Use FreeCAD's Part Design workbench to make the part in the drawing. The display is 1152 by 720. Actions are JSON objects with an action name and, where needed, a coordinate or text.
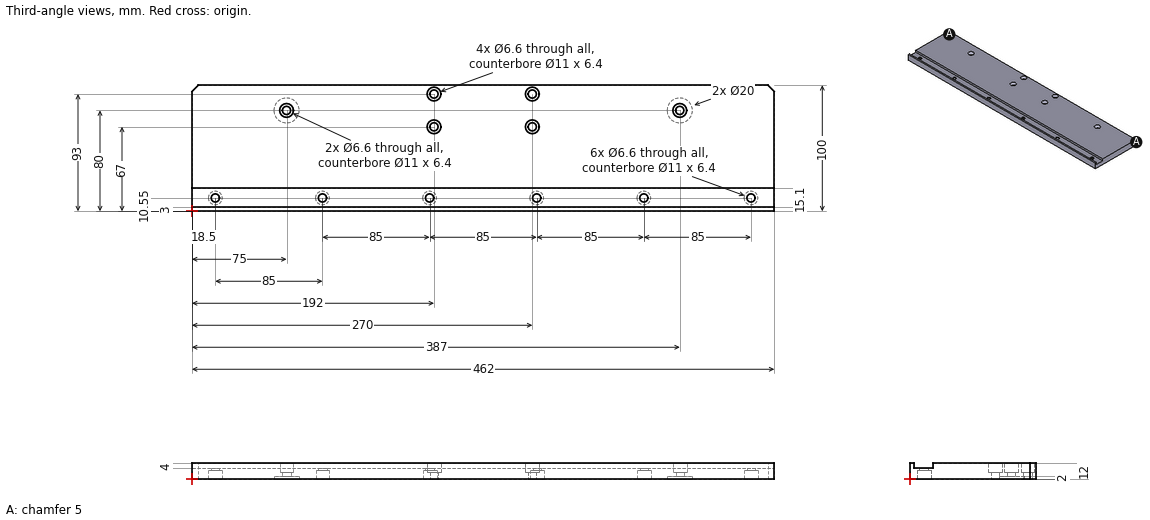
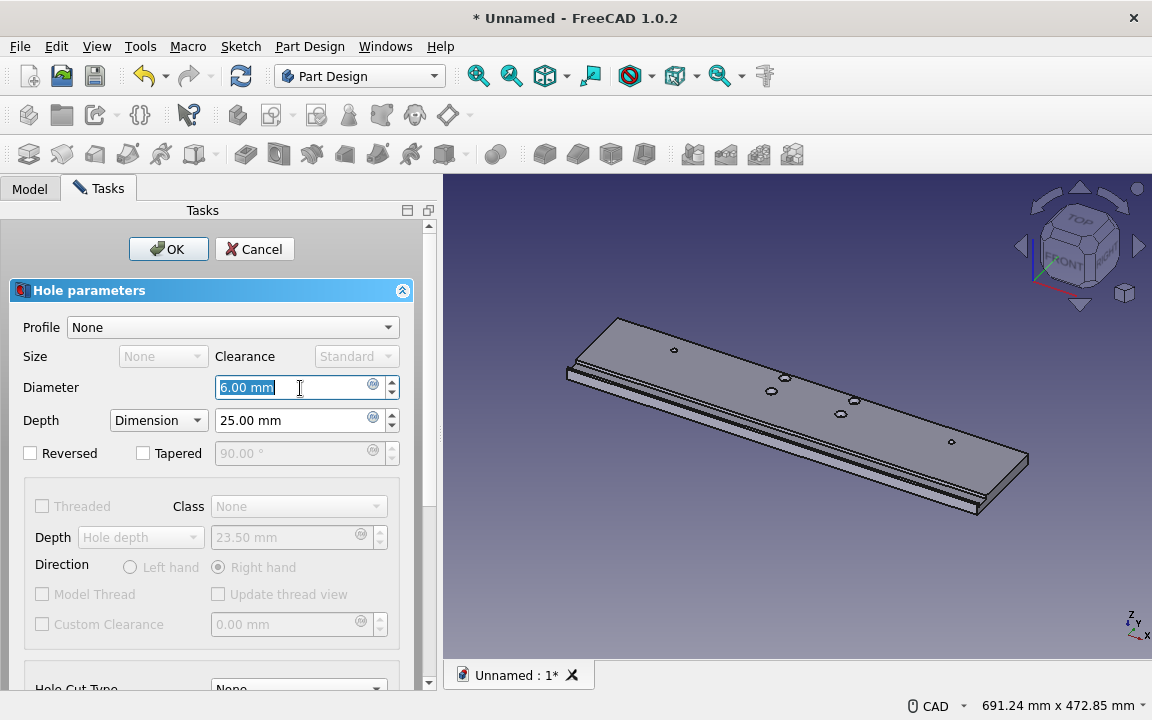
{"action": "type", "text": "6.6"}
{"action": "key", "text": "Tab"}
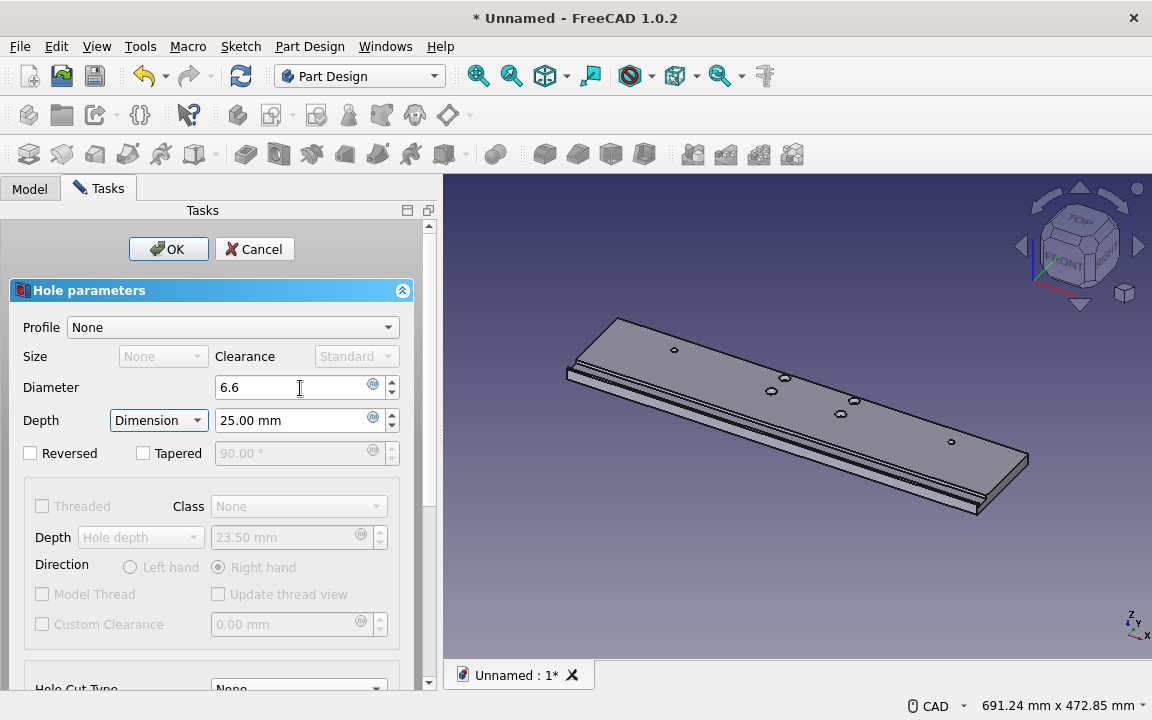
{"action": "left_click", "coordinate": [160, 420]}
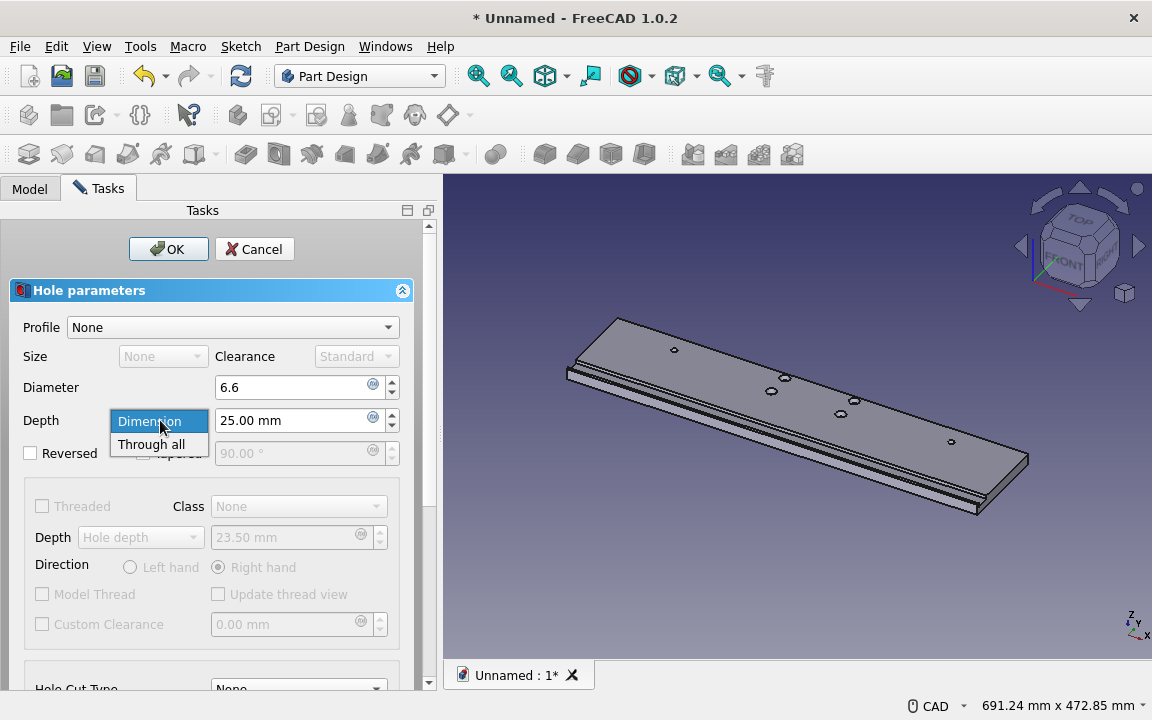
{"action": "left_click", "coordinate": [158, 444]}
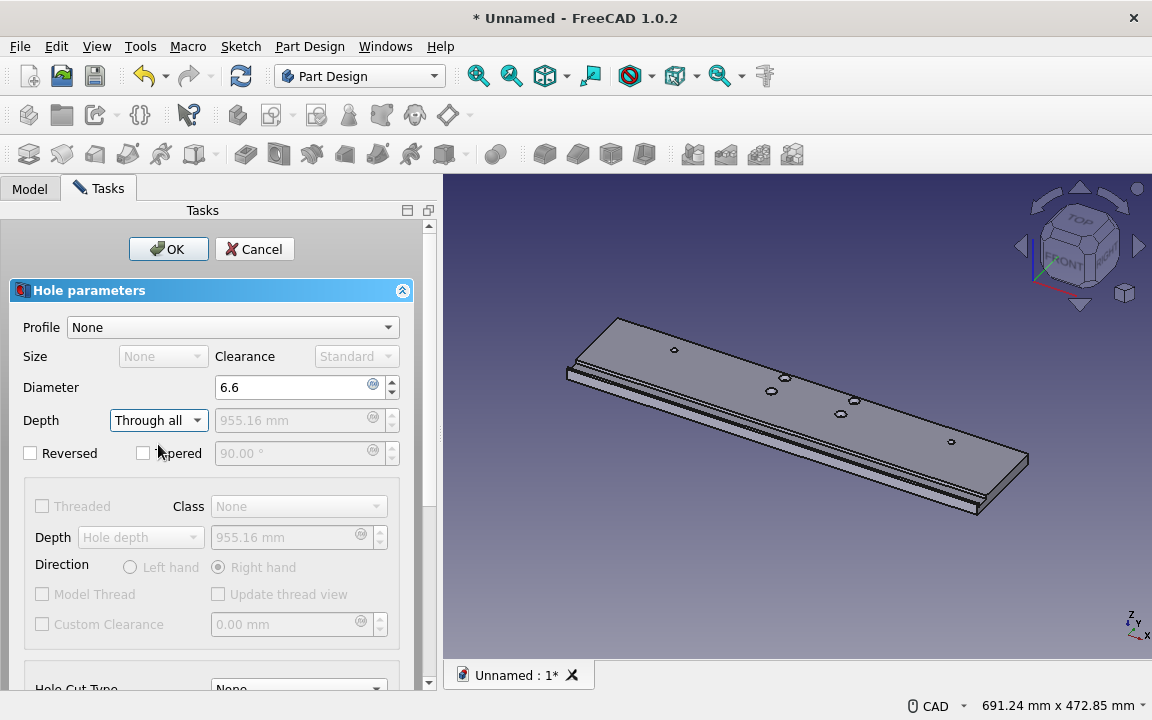
{"action": "scroll", "coordinate": [429, 455], "scroll_direction": "down", "scroll_amount": 2}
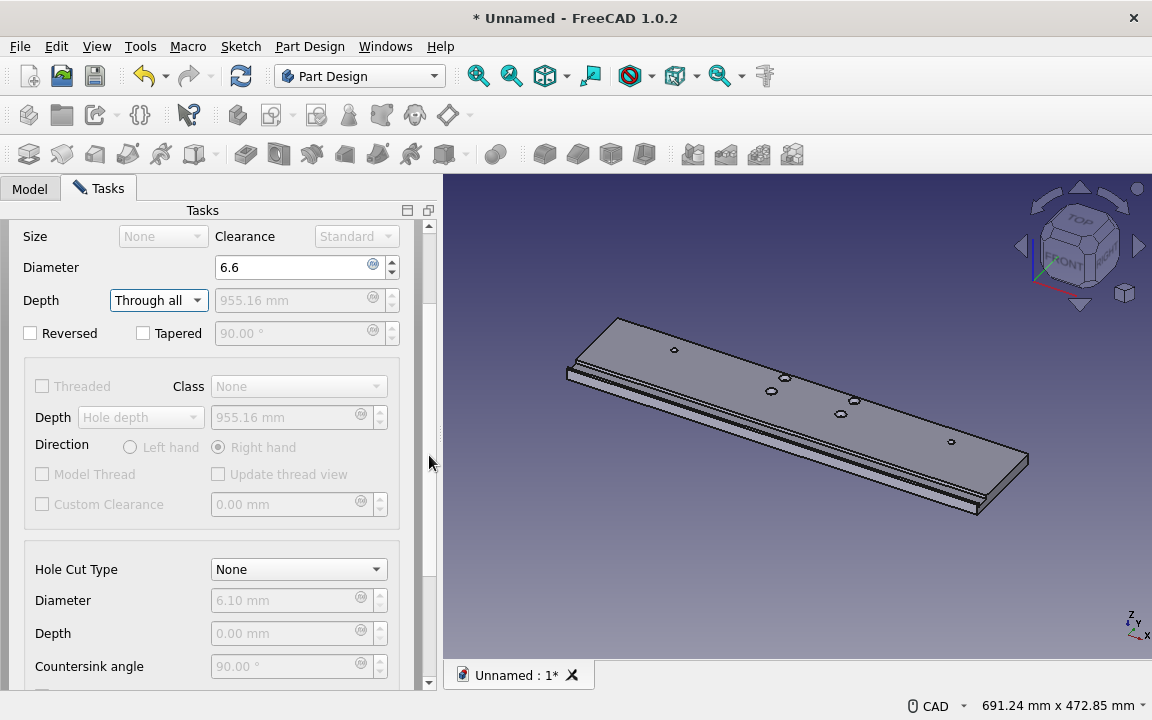
{"action": "left_click", "coordinate": [300, 570]}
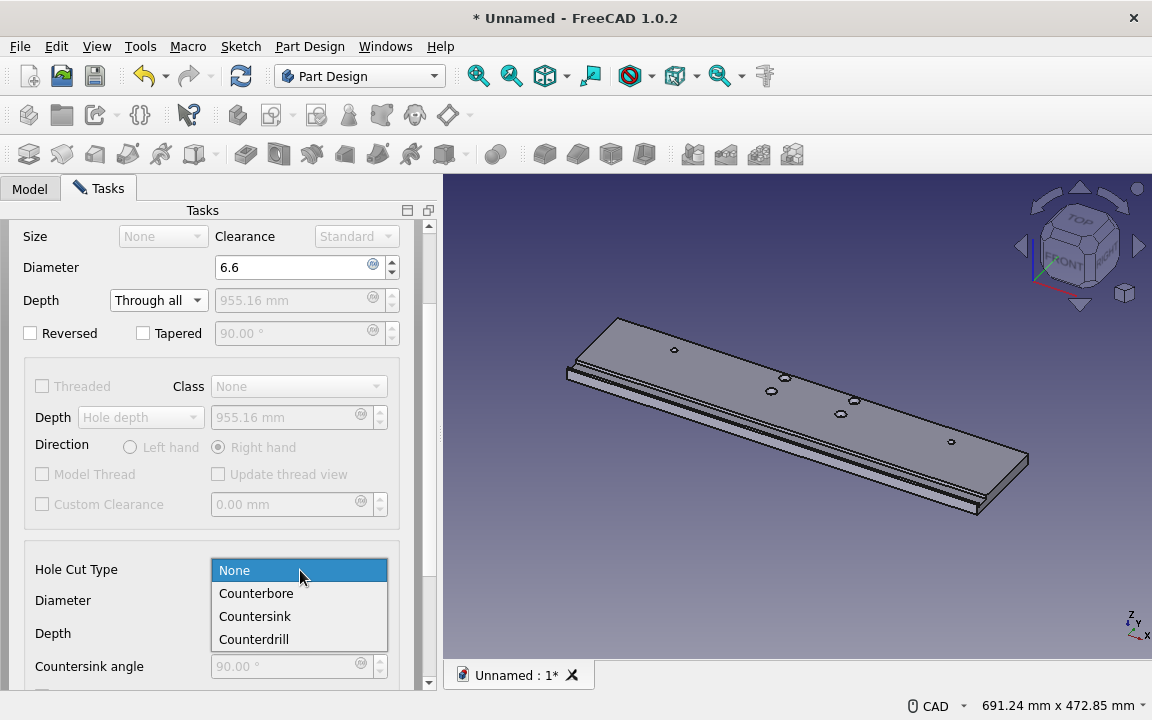
{"action": "left_click", "coordinate": [298, 594]}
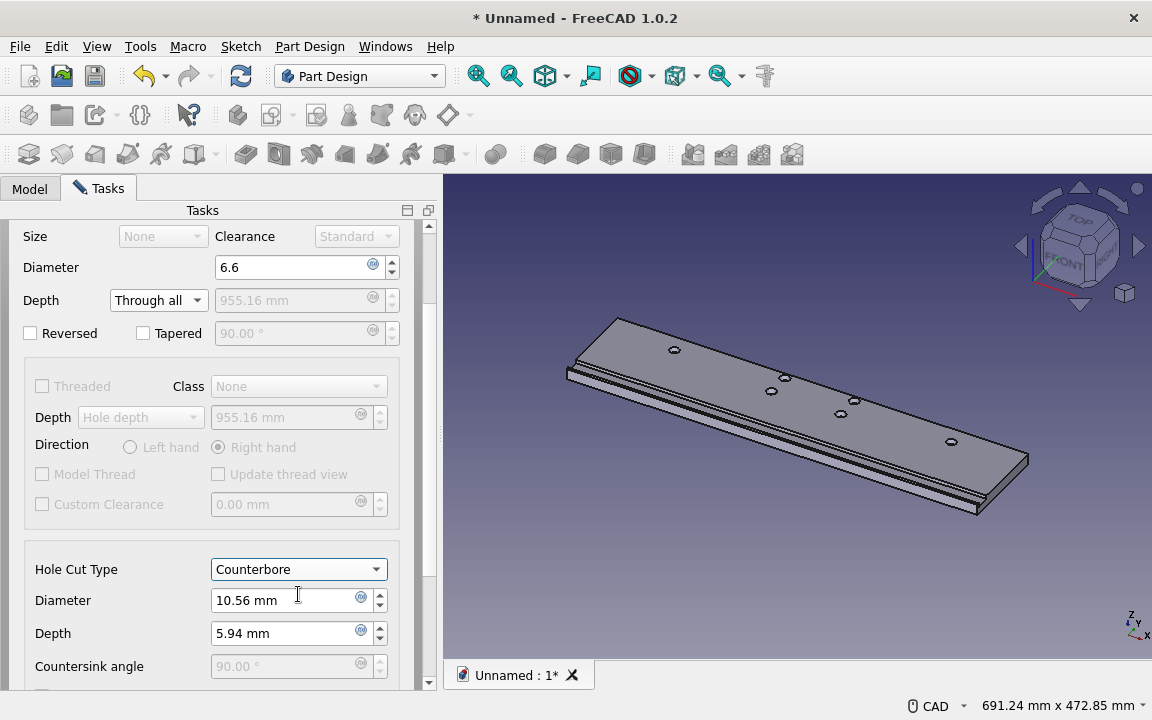
{"action": "triple_click", "coordinate": [292, 600]}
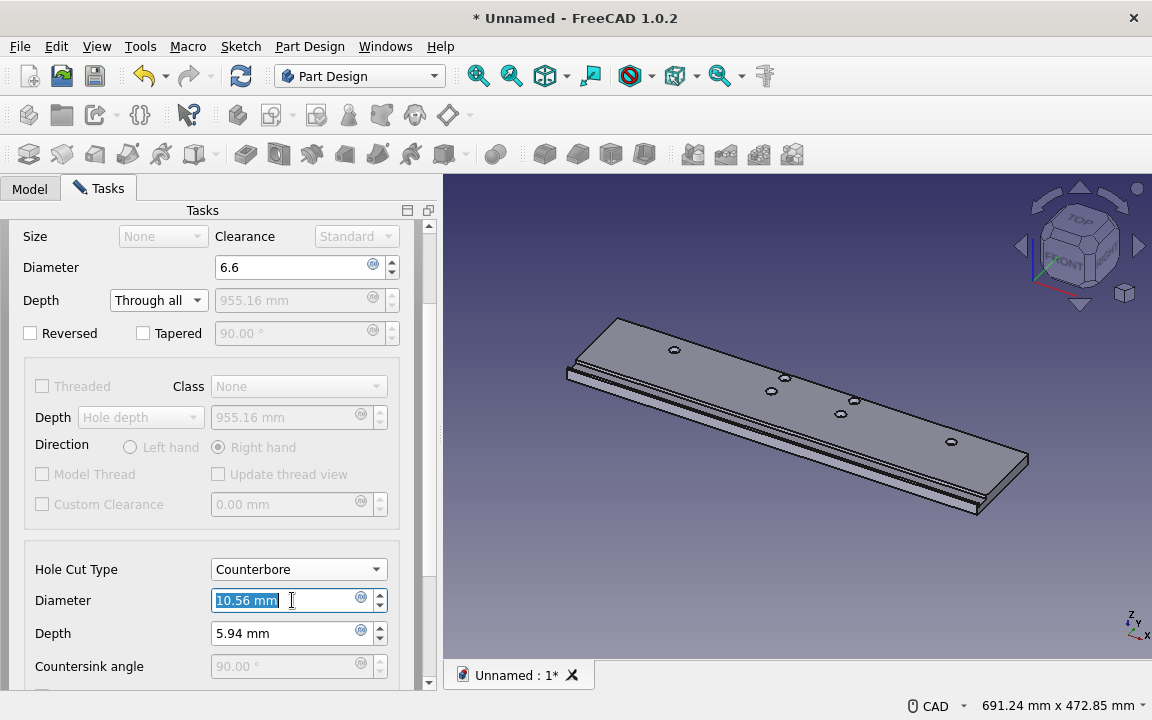
{"action": "type", "text": "11"}
{"action": "key", "text": "Tab"}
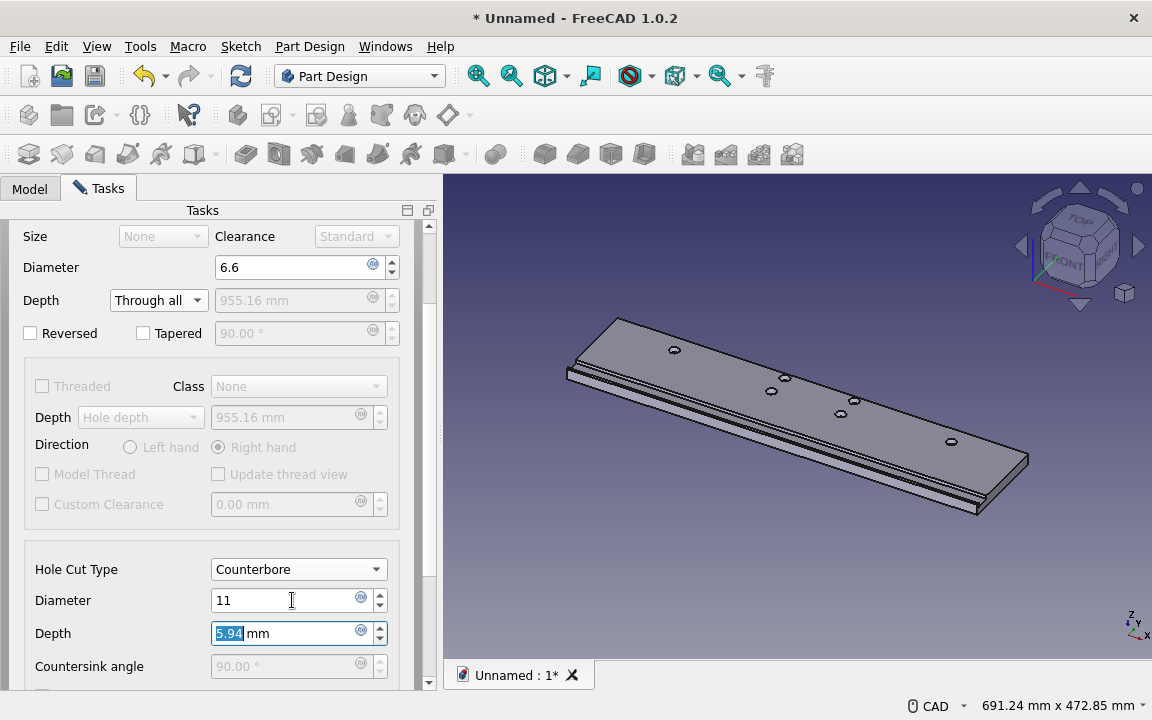
{"action": "type", "text": "6.4"}
{"action": "key", "text": "Tab"}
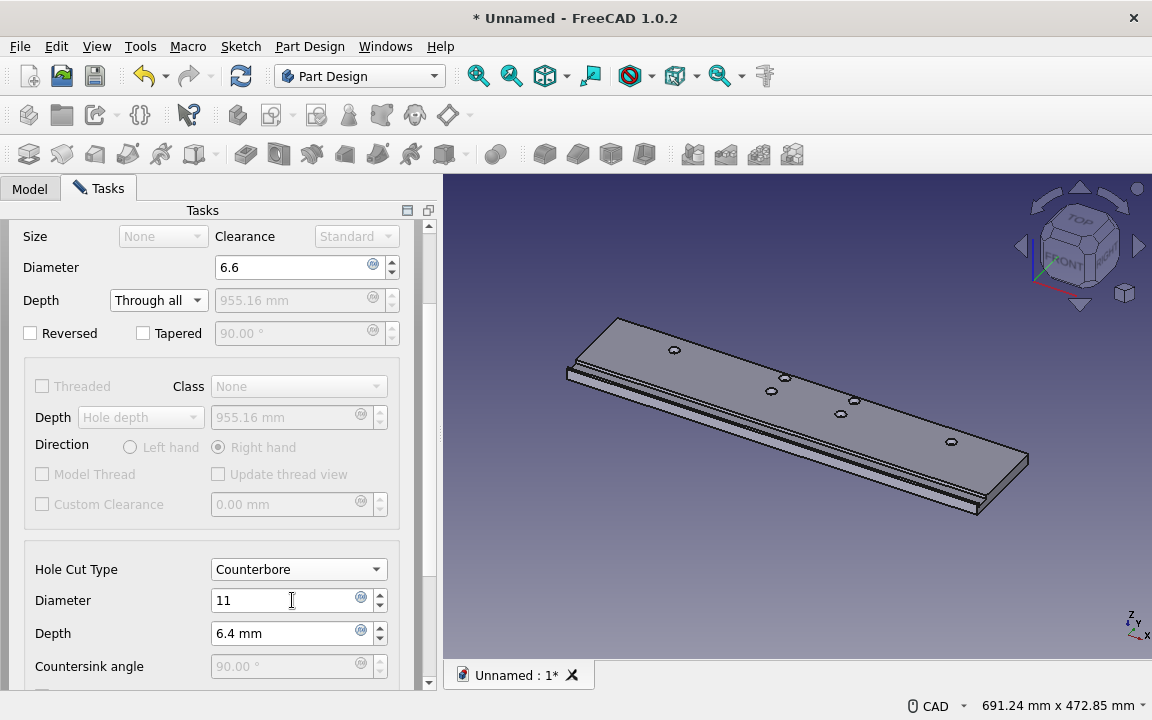
{"action": "scroll", "coordinate": [429, 455], "scroll_direction": "up", "scroll_amount": 3}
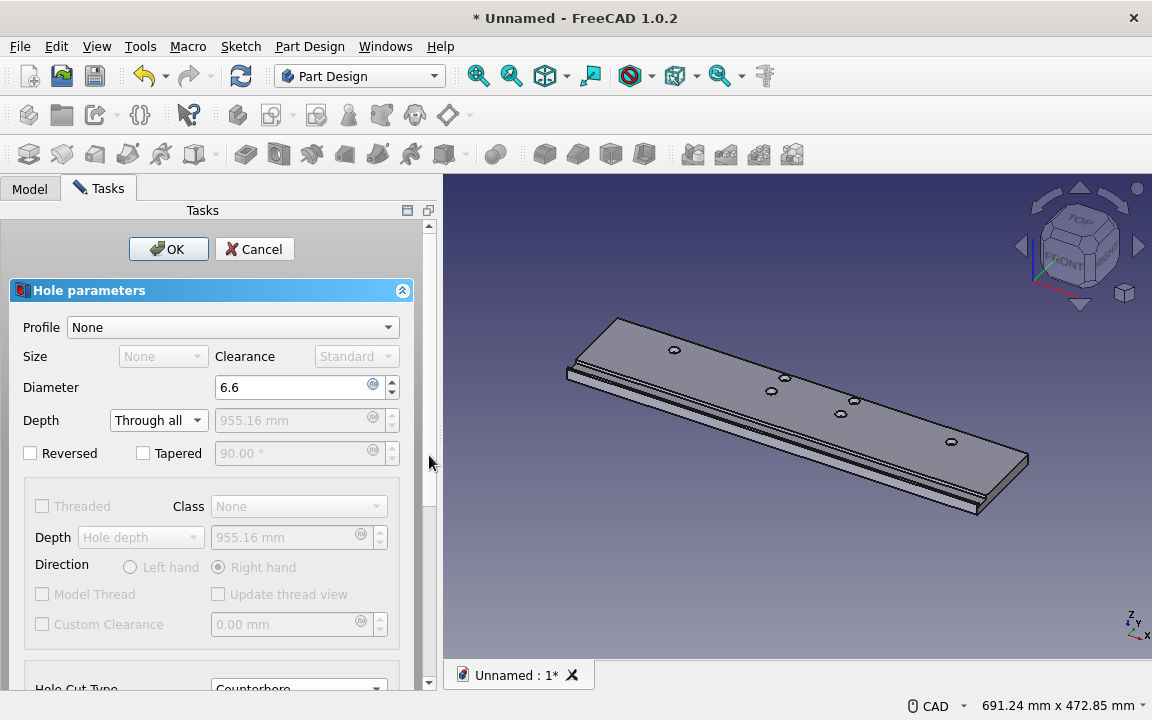
{"action": "left_click", "coordinate": [169, 249]}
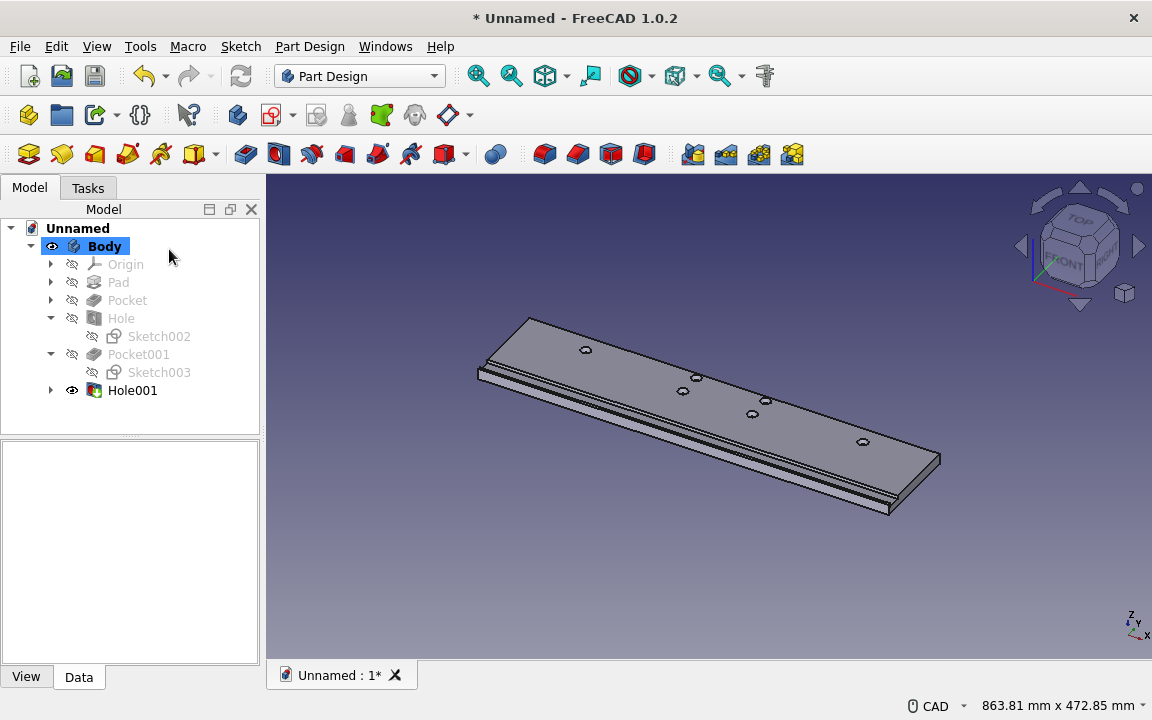
{"action": "left_click", "coordinate": [270, 116]}